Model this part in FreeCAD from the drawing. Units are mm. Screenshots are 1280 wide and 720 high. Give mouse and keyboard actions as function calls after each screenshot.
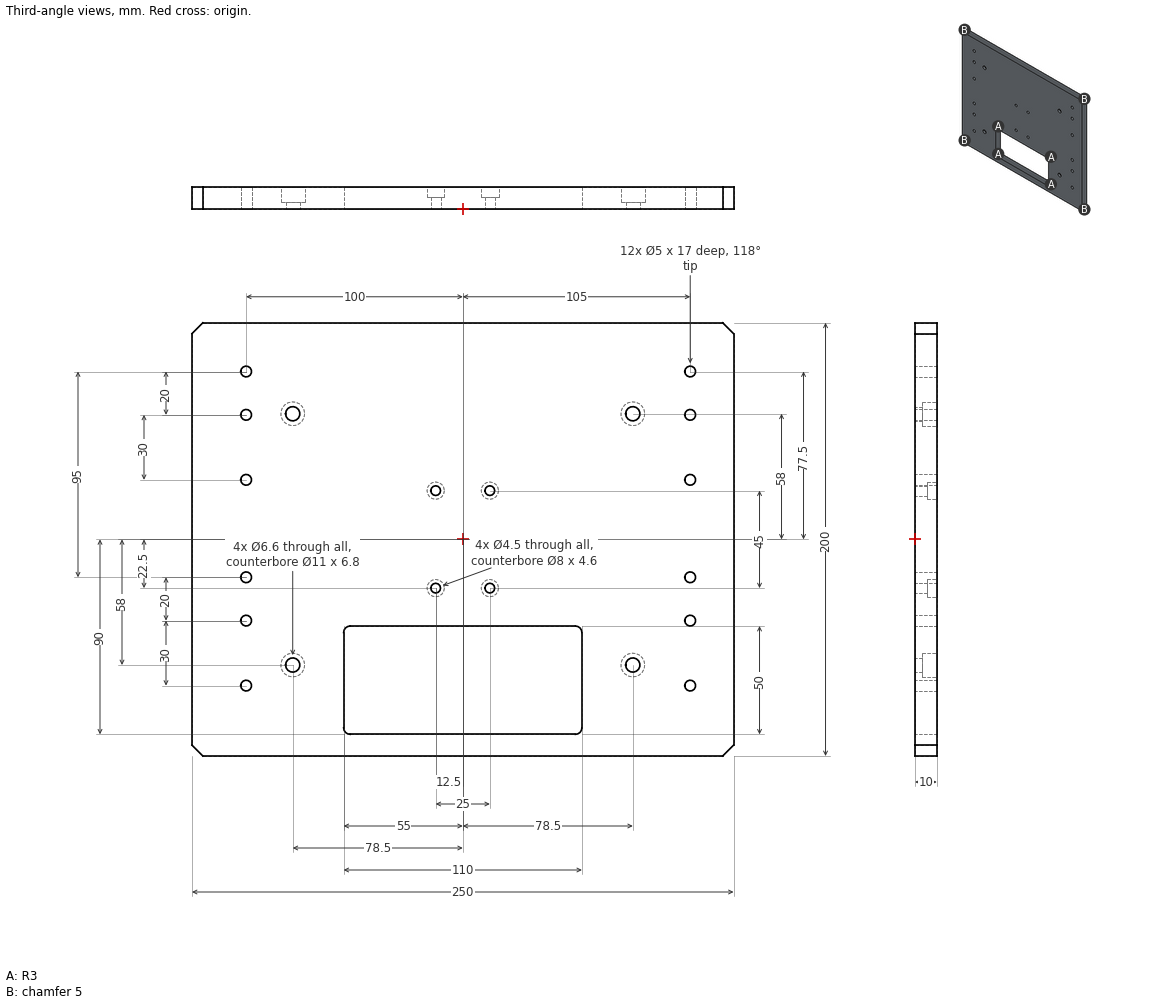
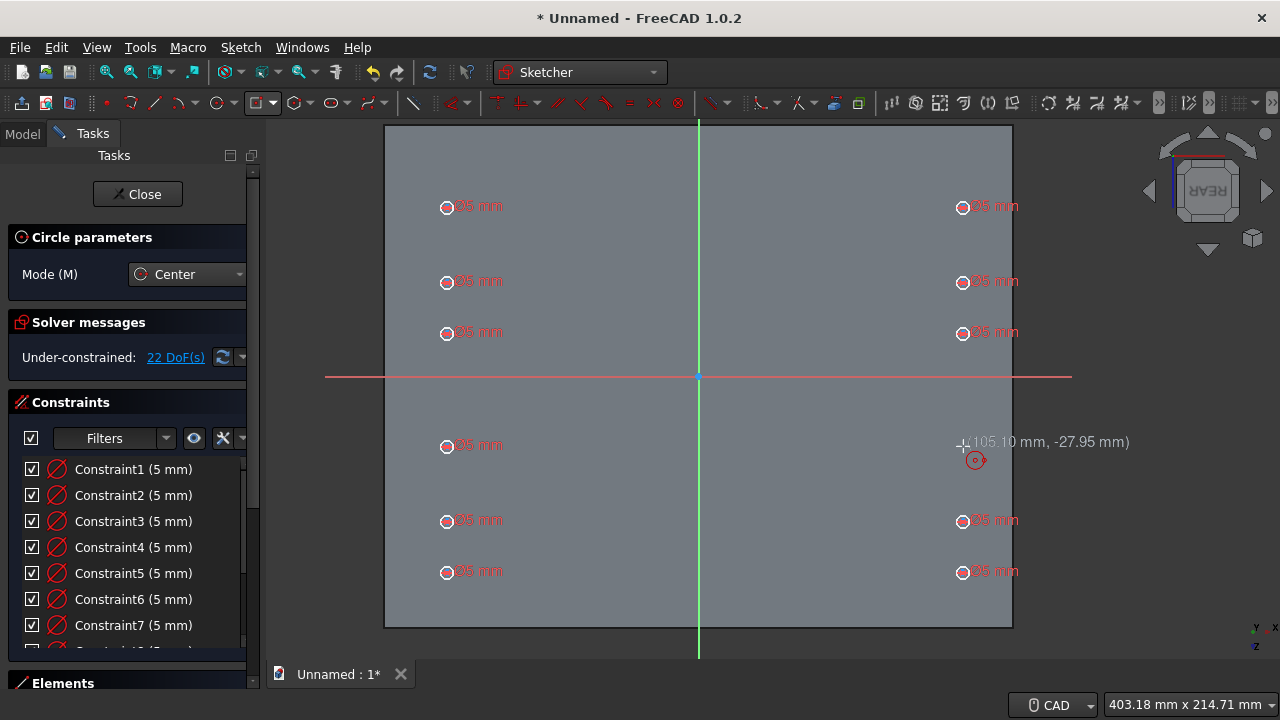
click(963, 446)
move(967, 441)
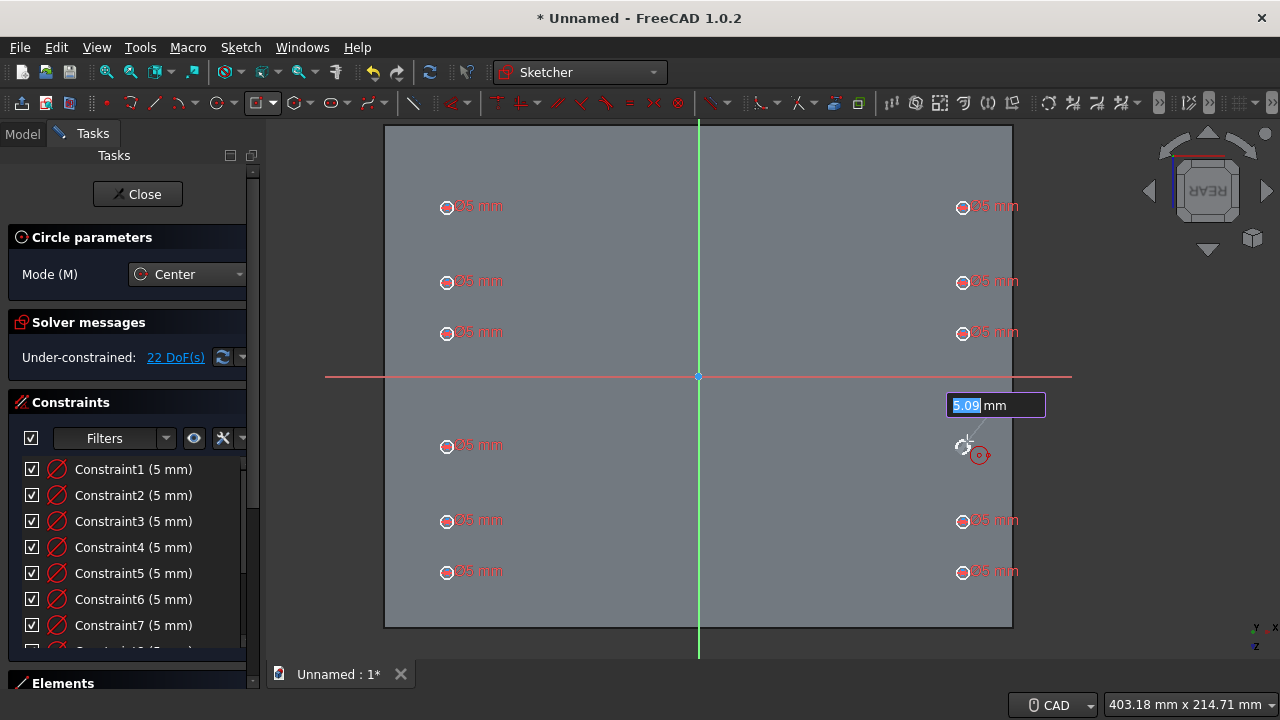
text(5)
key(Return)
key(Escape)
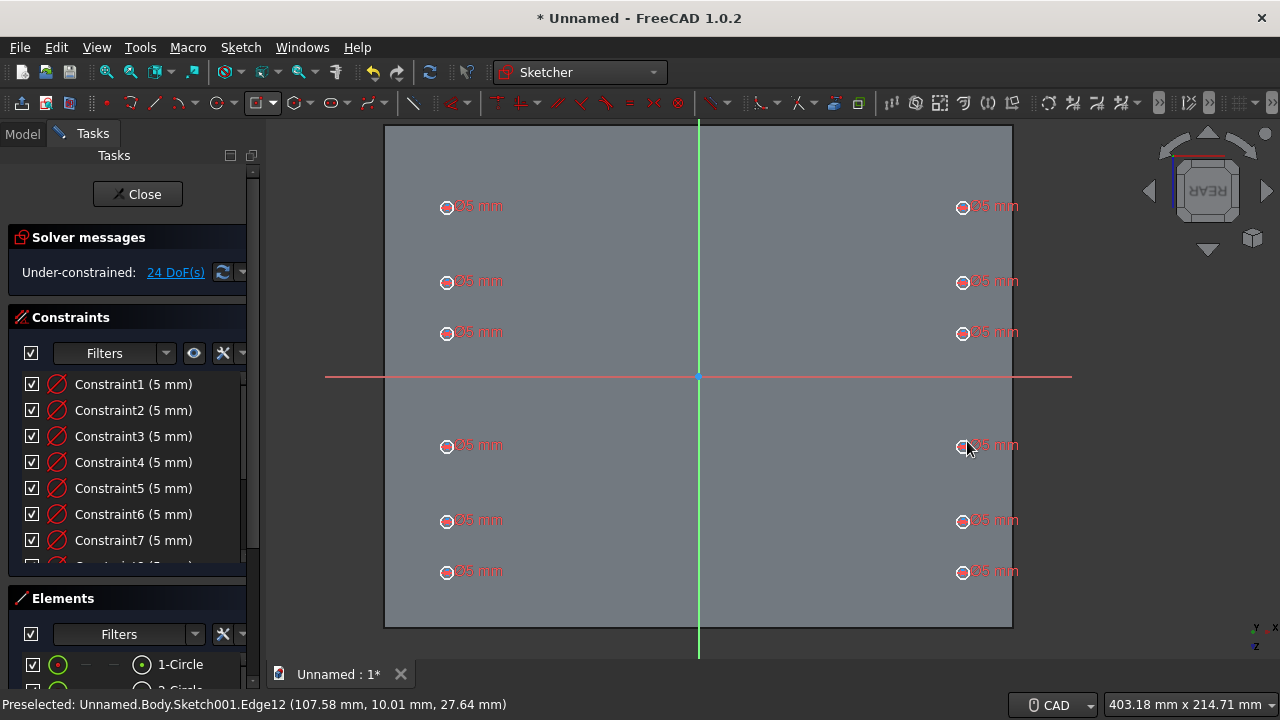
click(963, 573)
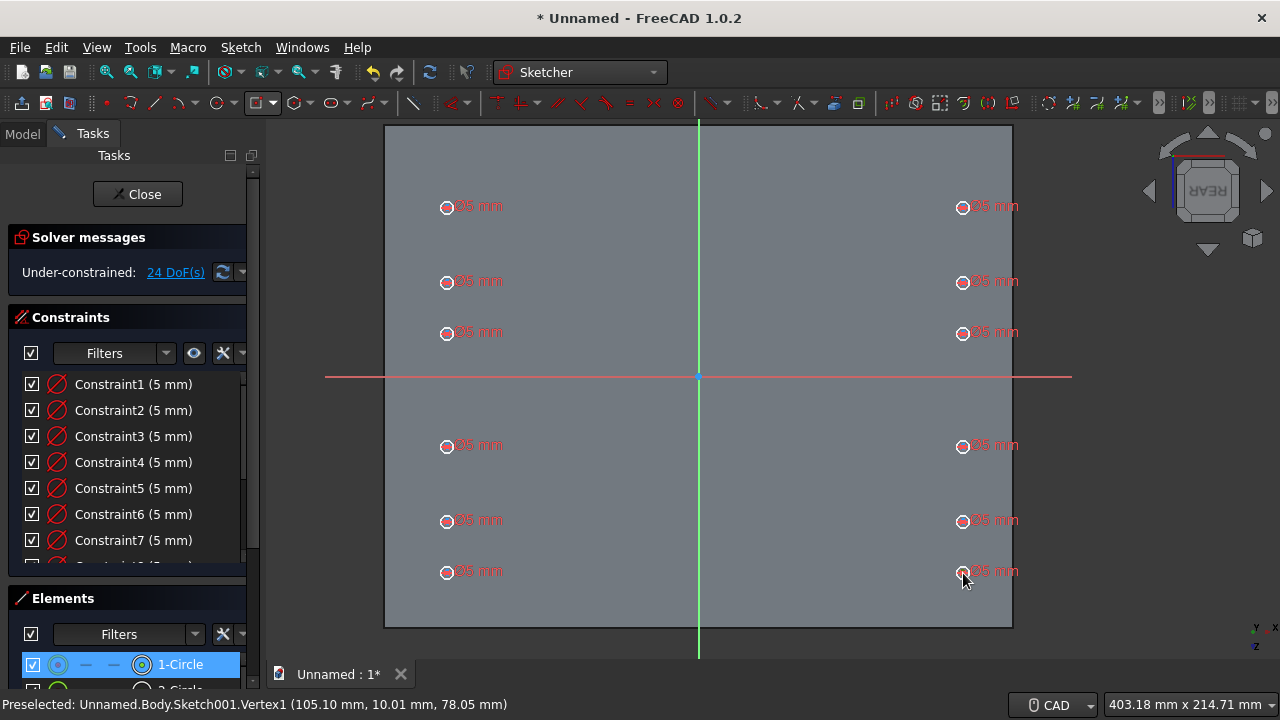
click(447, 573)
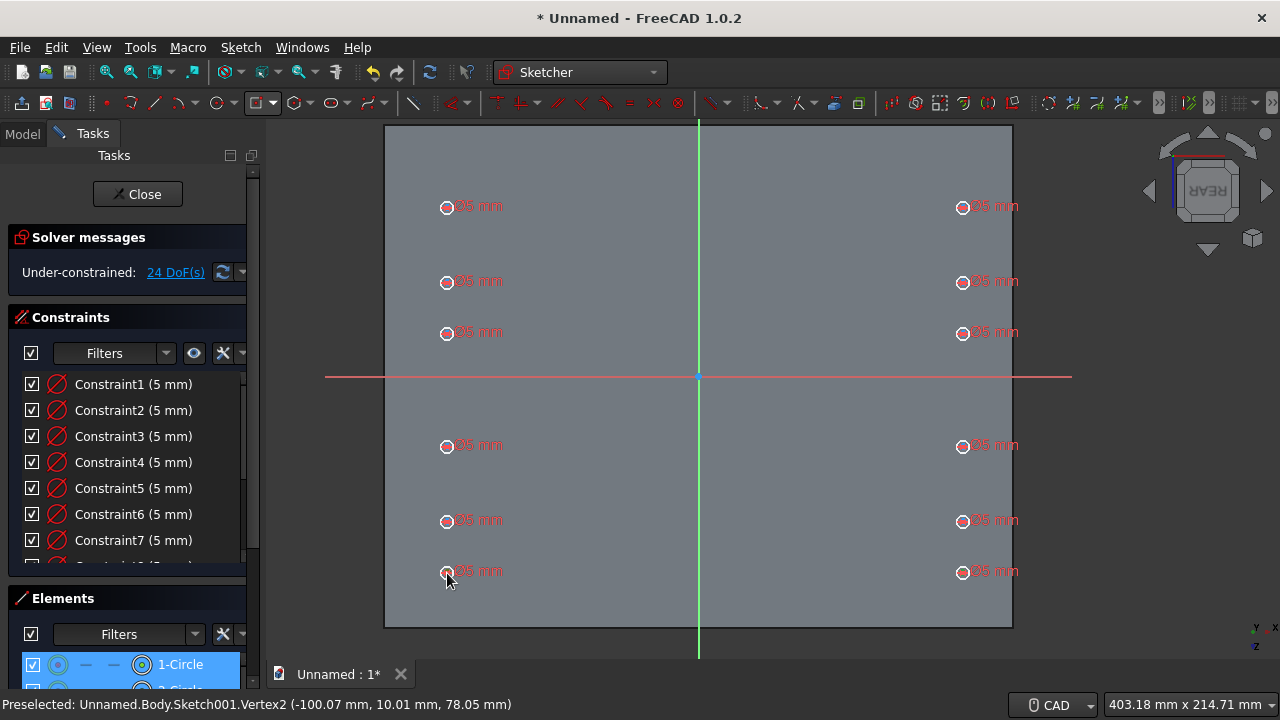
key(h)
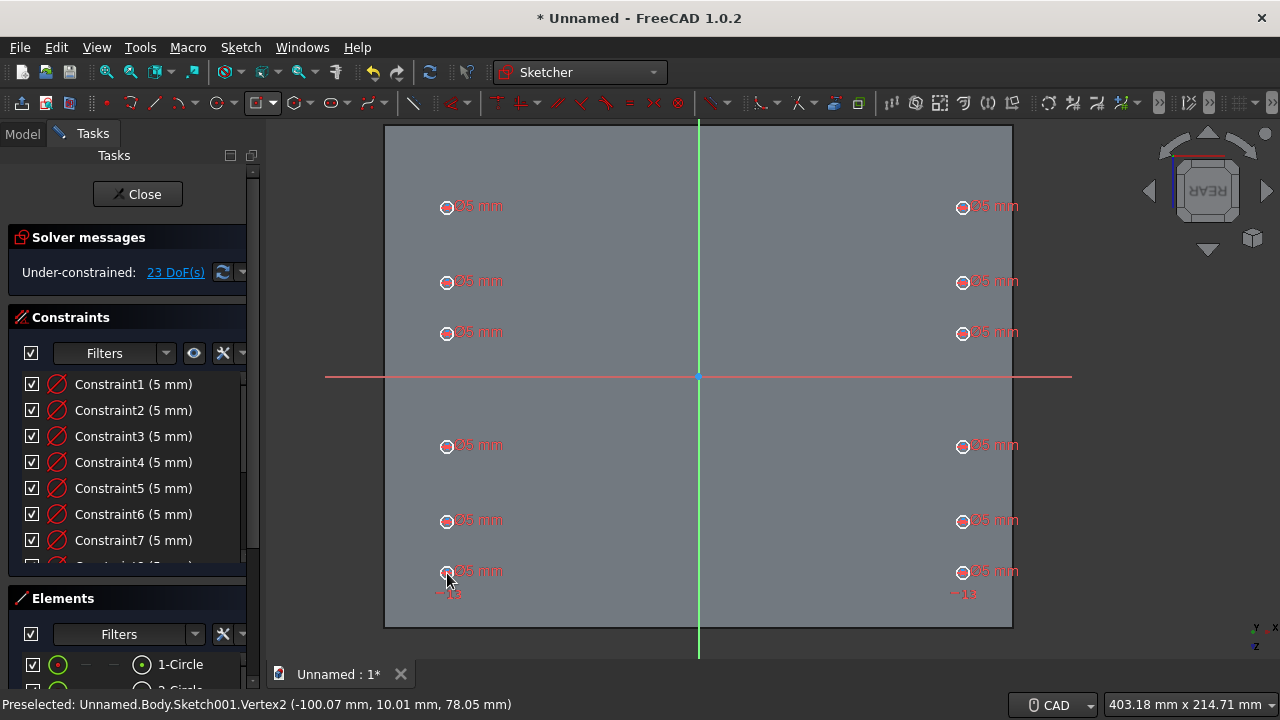
click(447, 573)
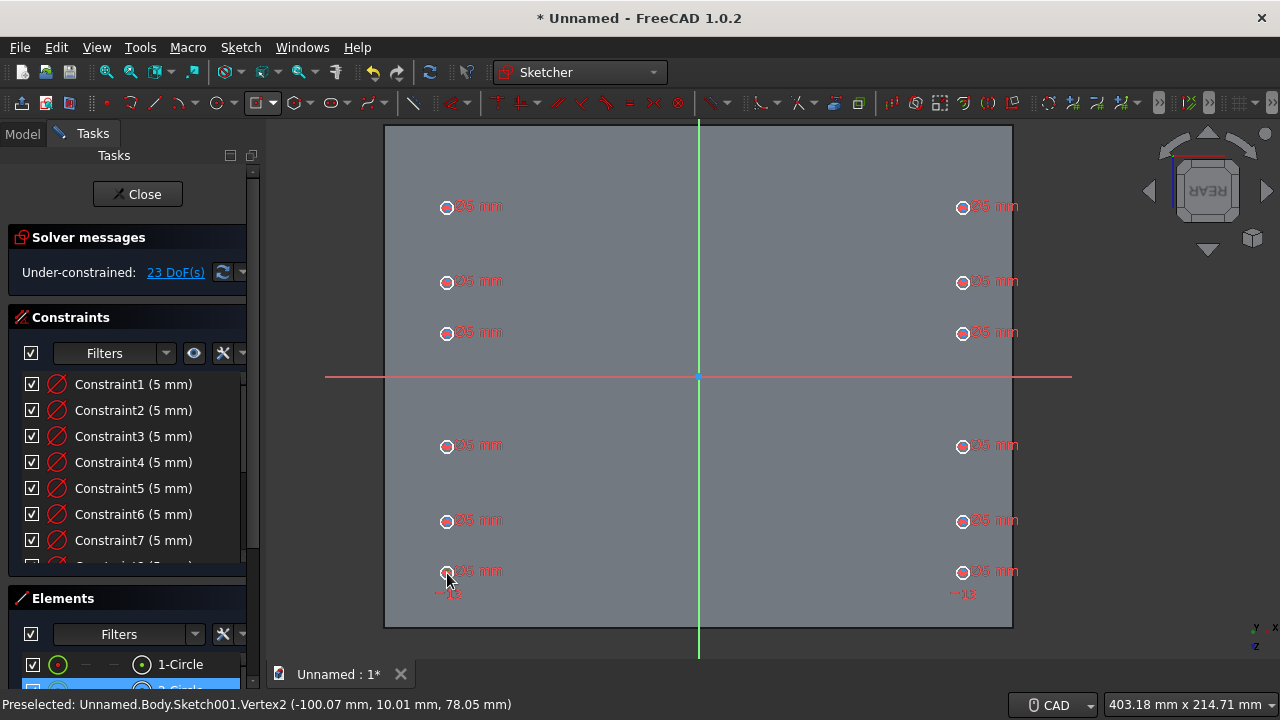
click(447, 334)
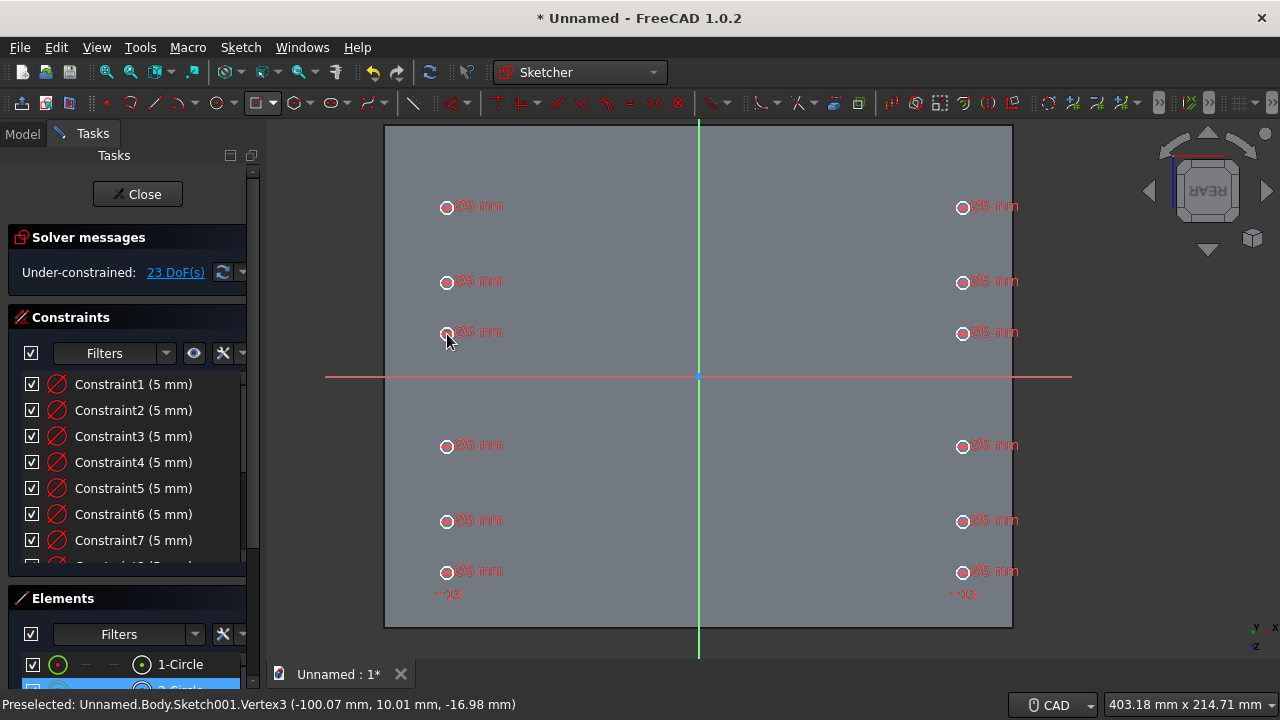
click(540, 104)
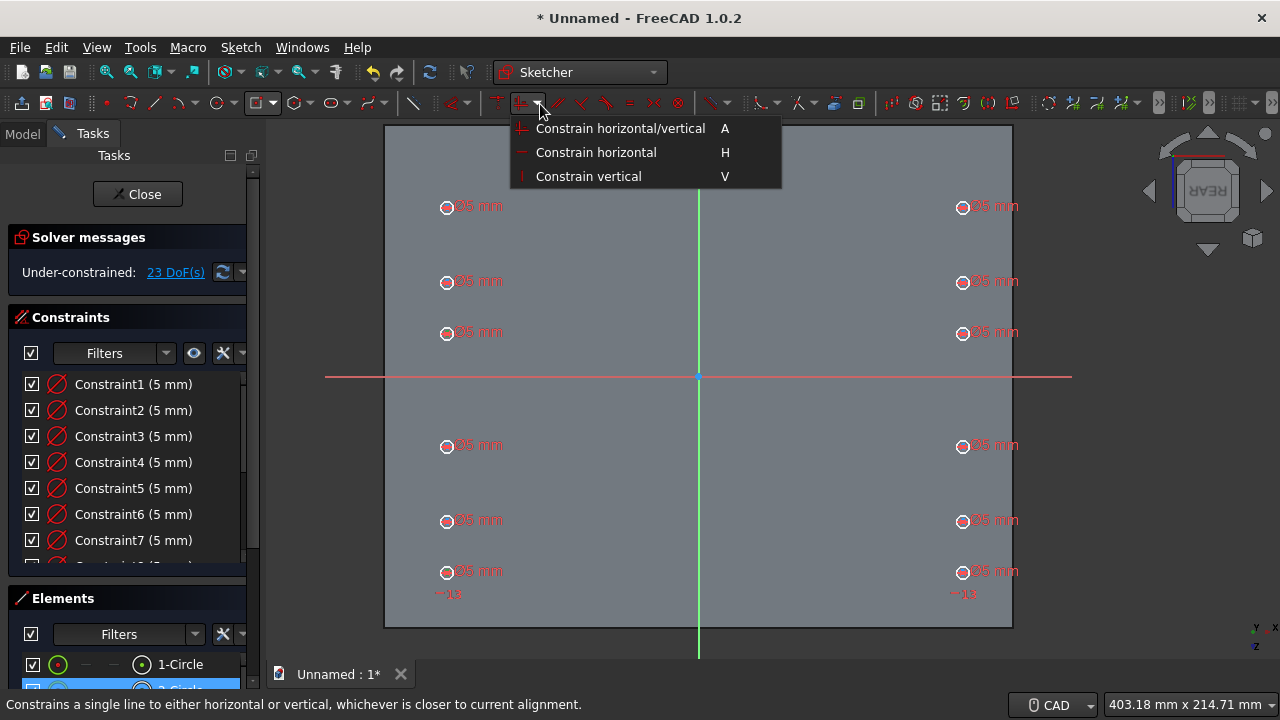
click(646, 176)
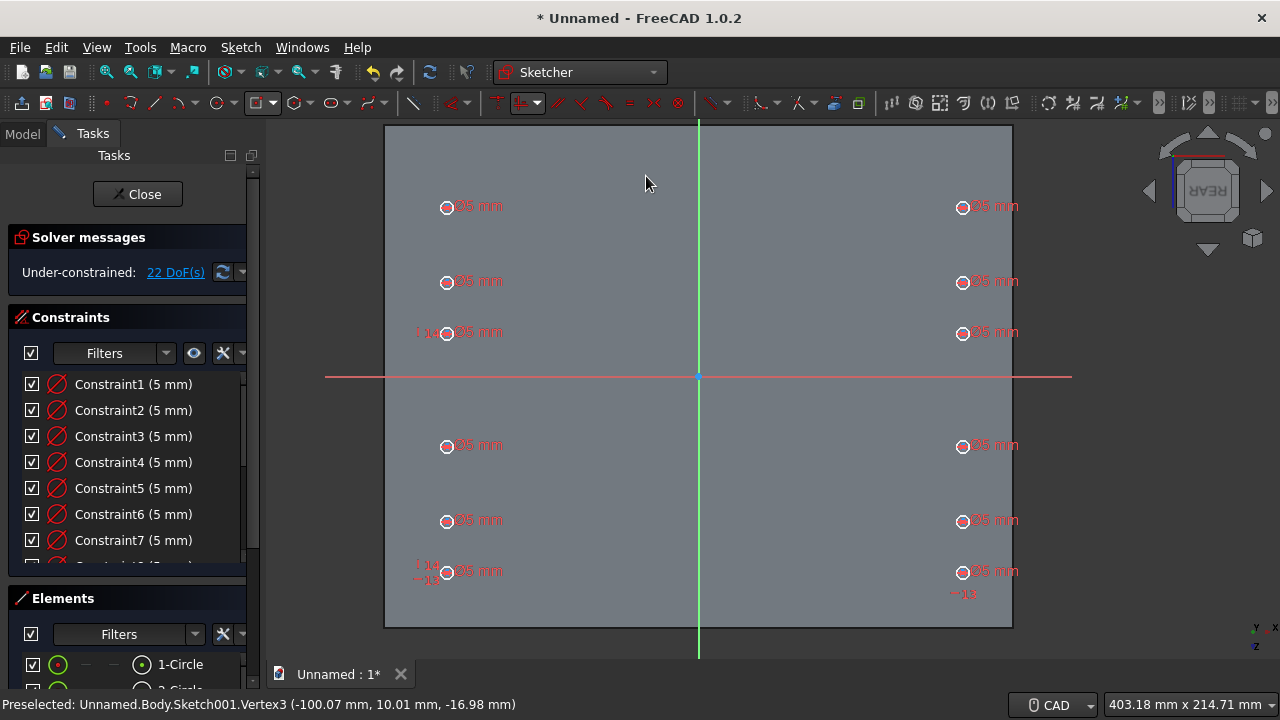
click(963, 573)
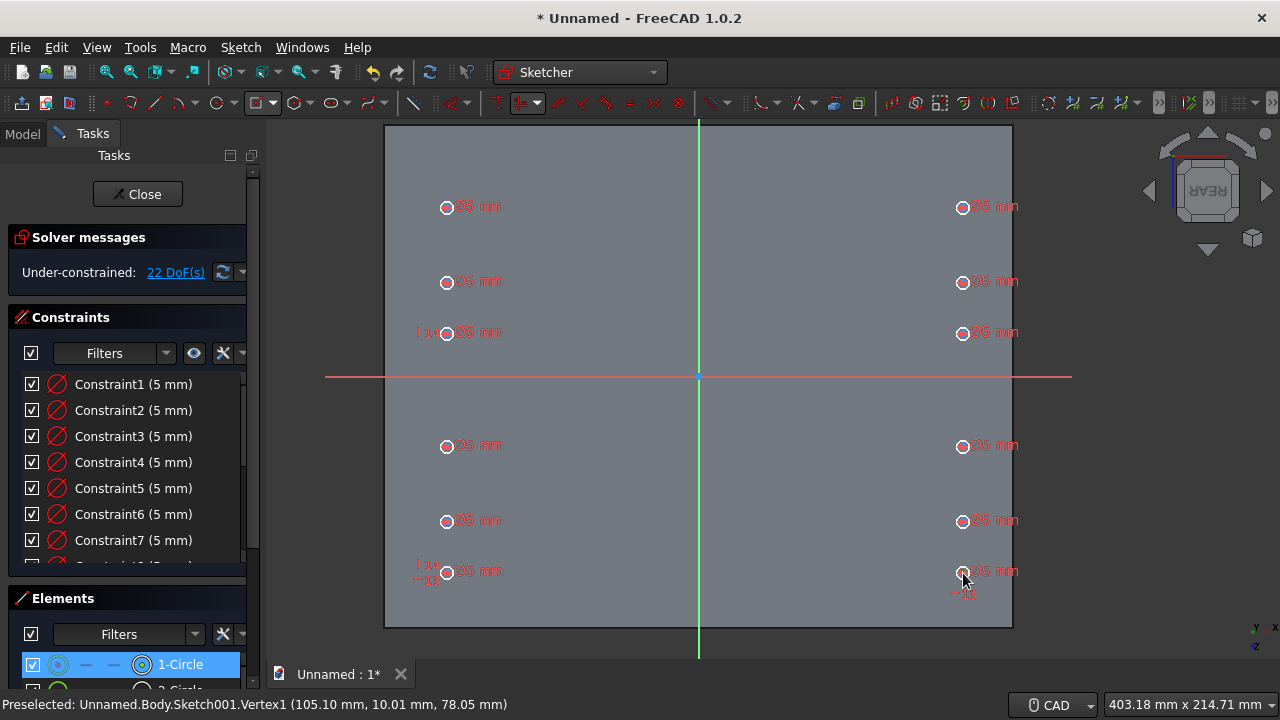
click(963, 334)